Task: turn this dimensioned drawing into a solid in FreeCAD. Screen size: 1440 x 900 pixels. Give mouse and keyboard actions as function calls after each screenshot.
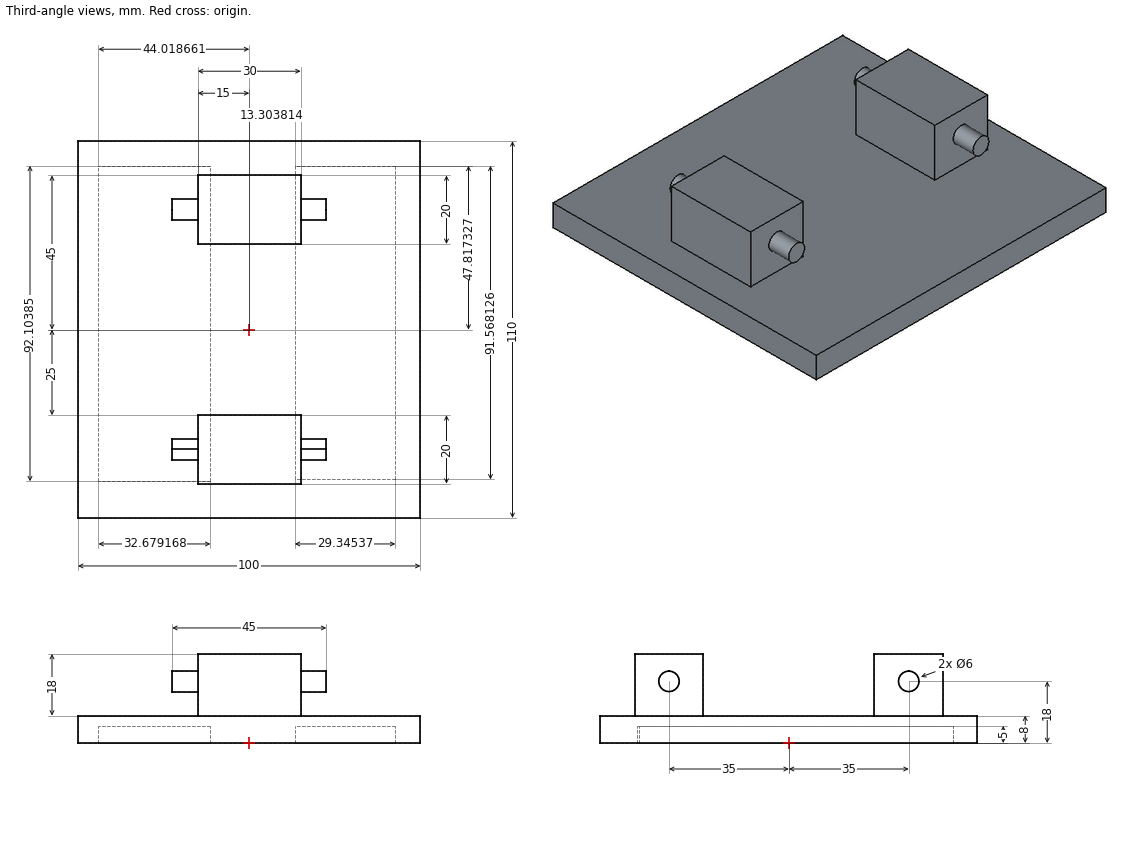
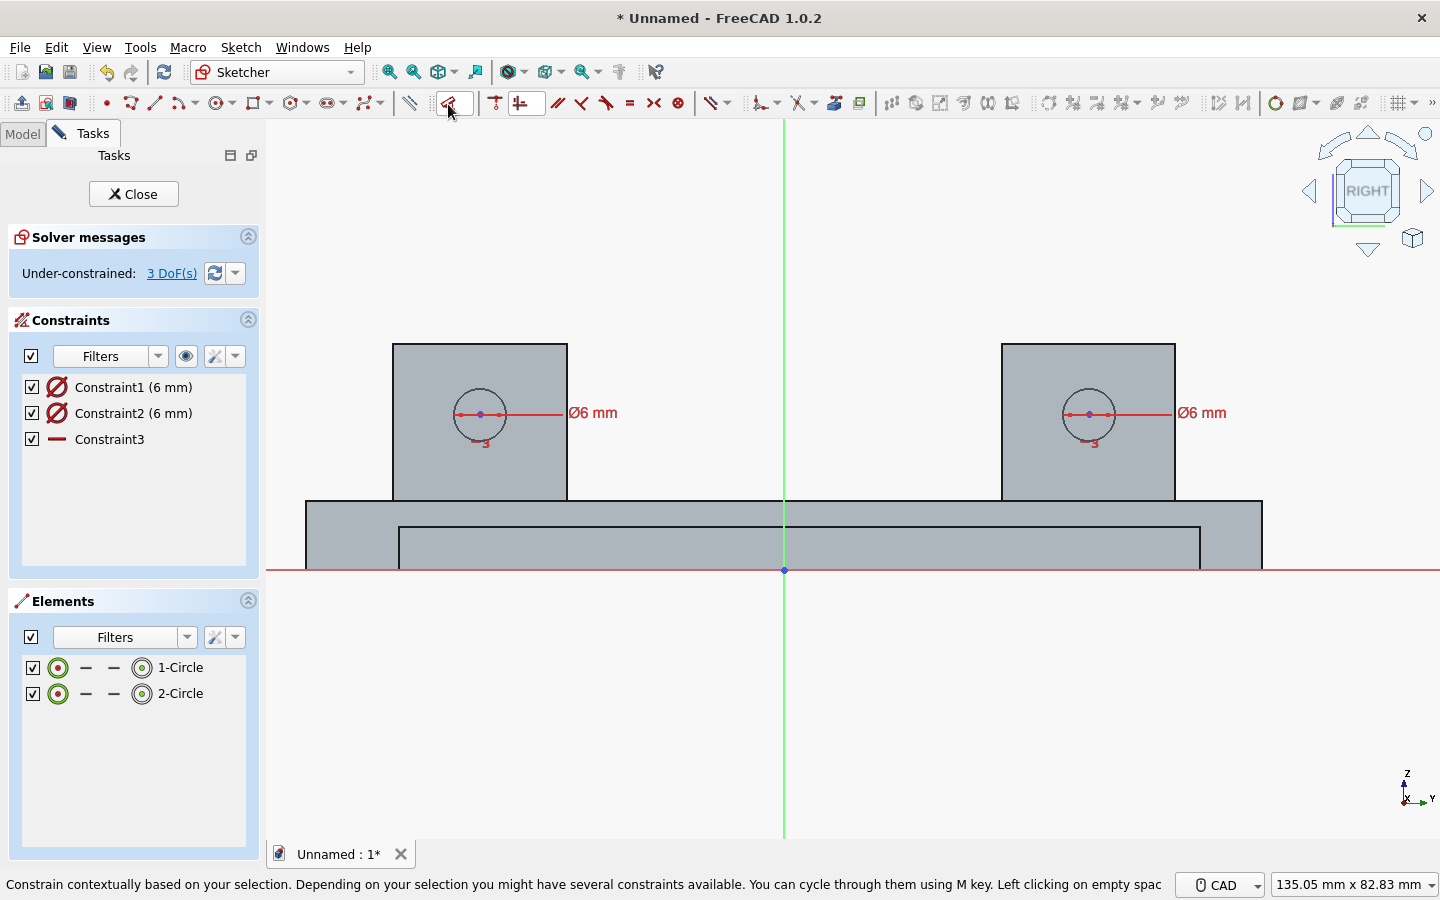
click(1089, 415)
click(937, 604)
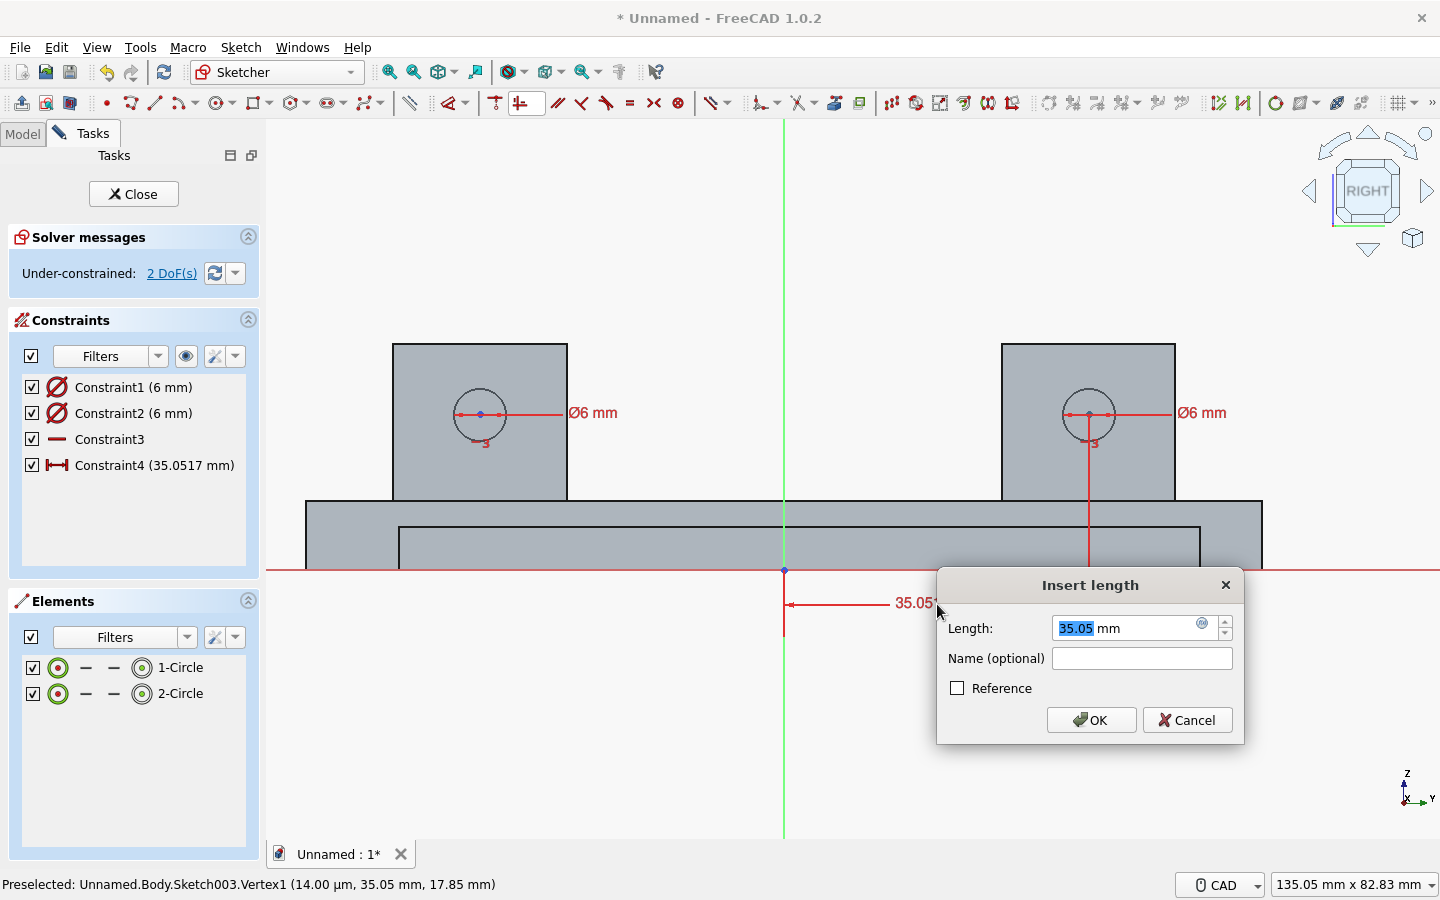
text(35)
key(Return)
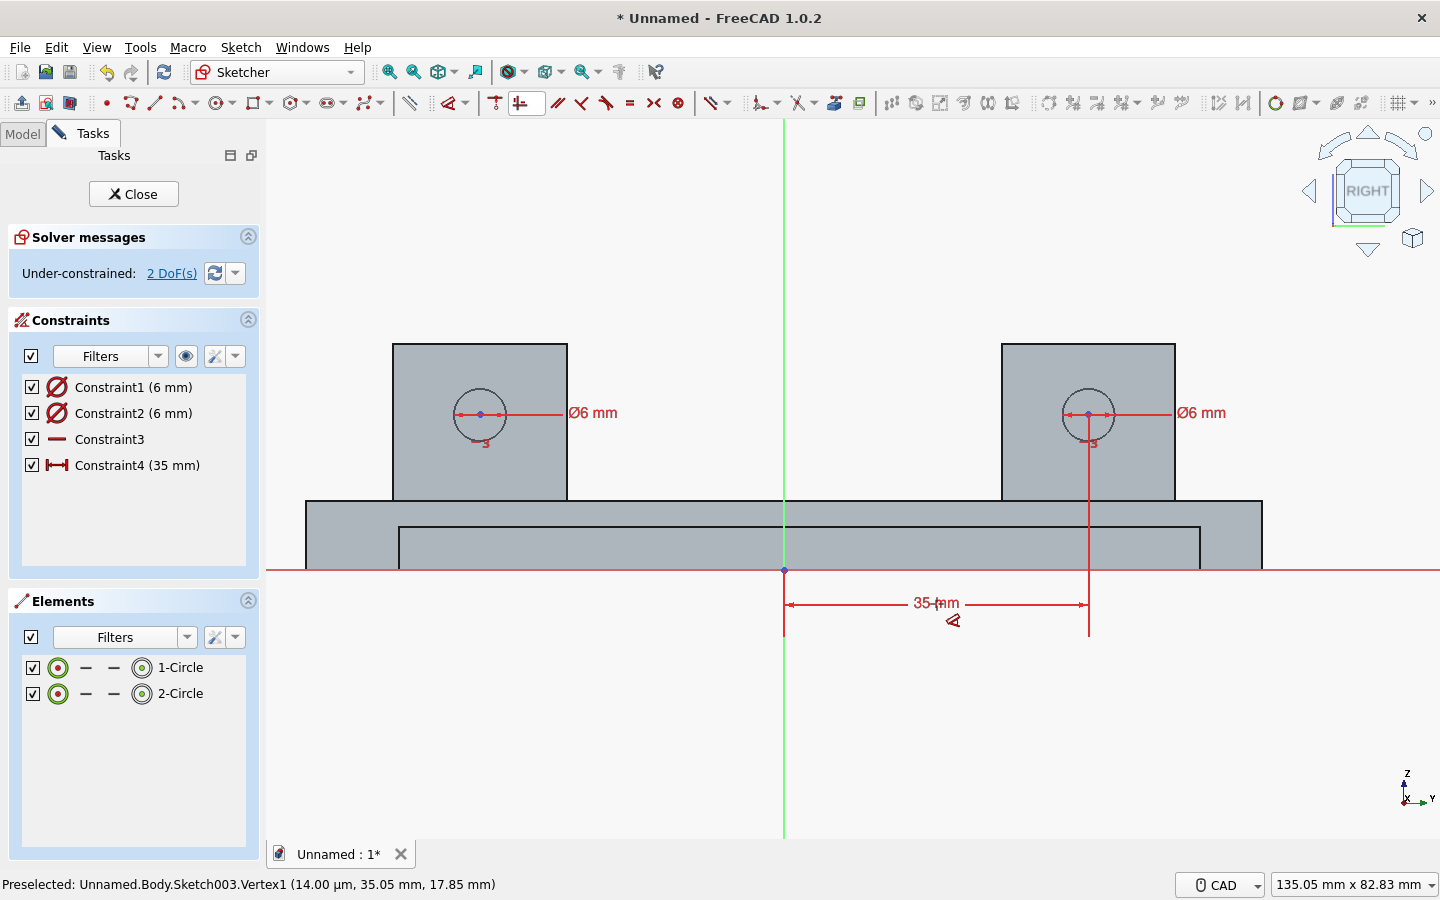
click(1089, 415)
click(1123, 493)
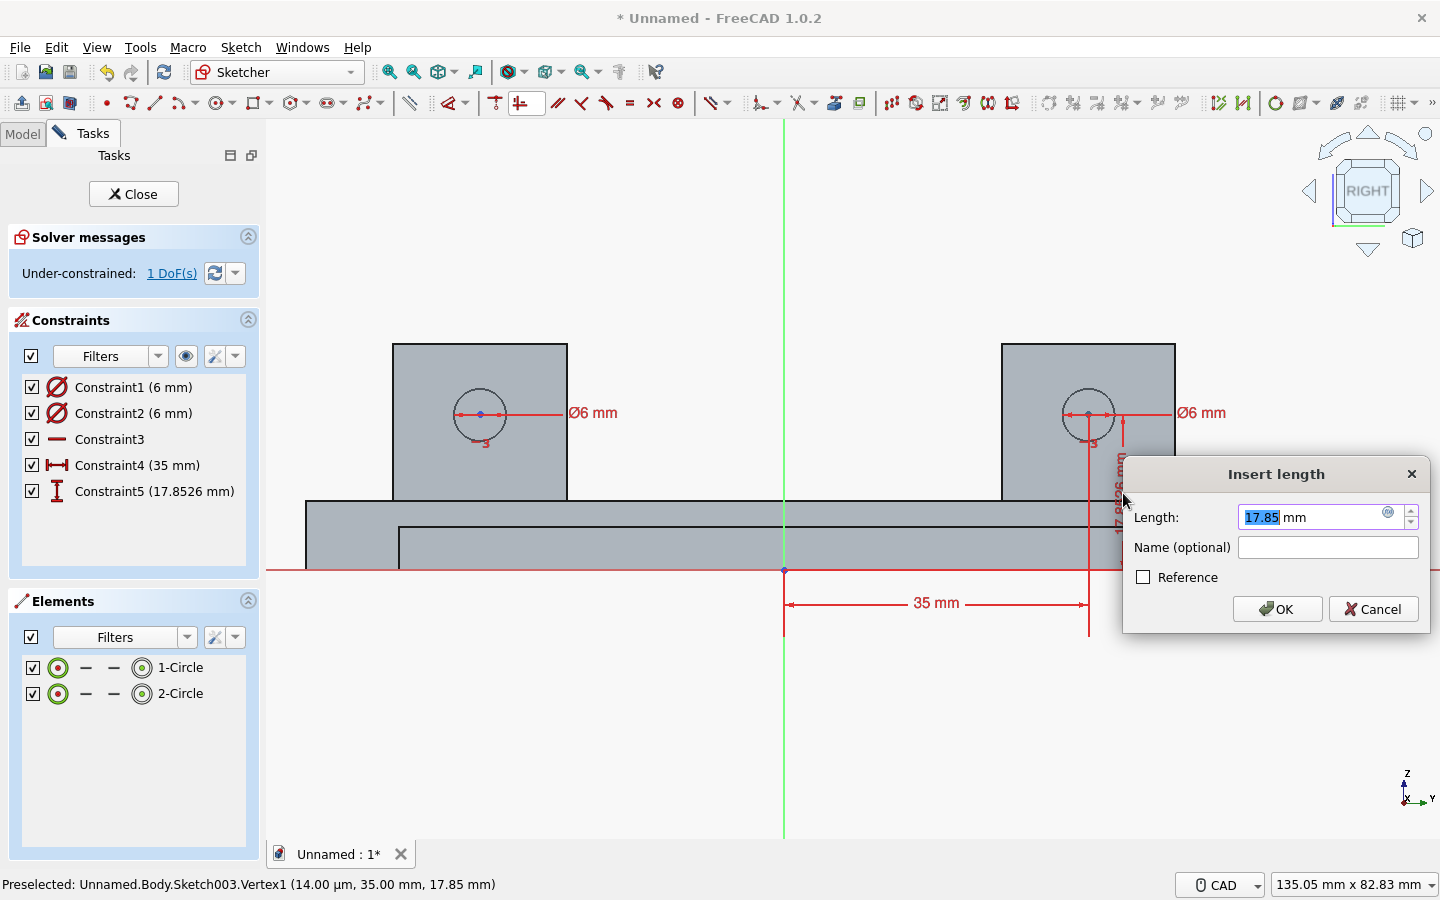
text(18)
key(Return)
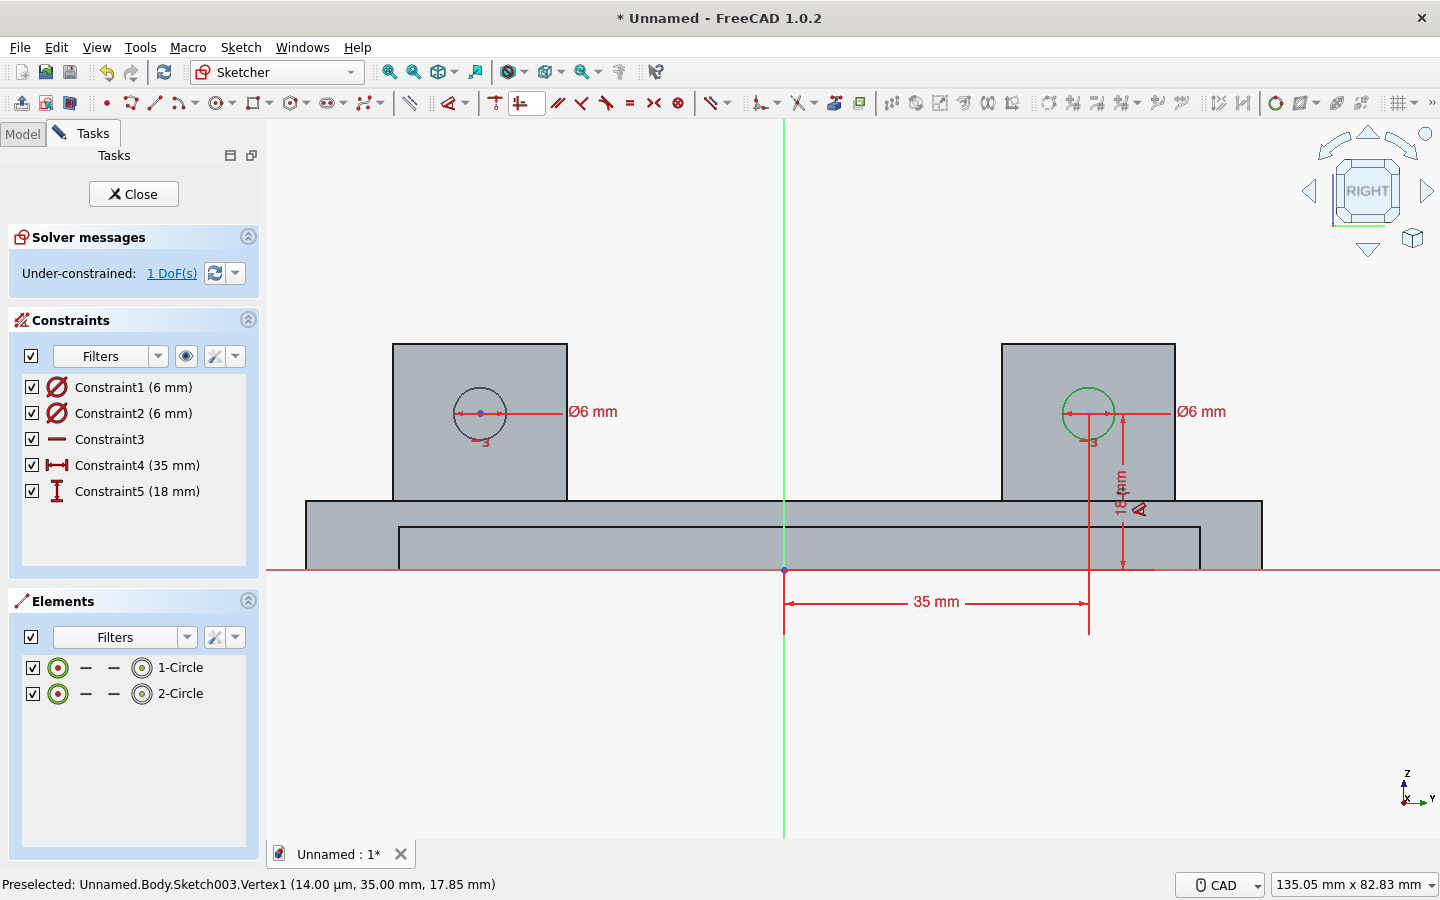
click(480, 414)
click(632, 604)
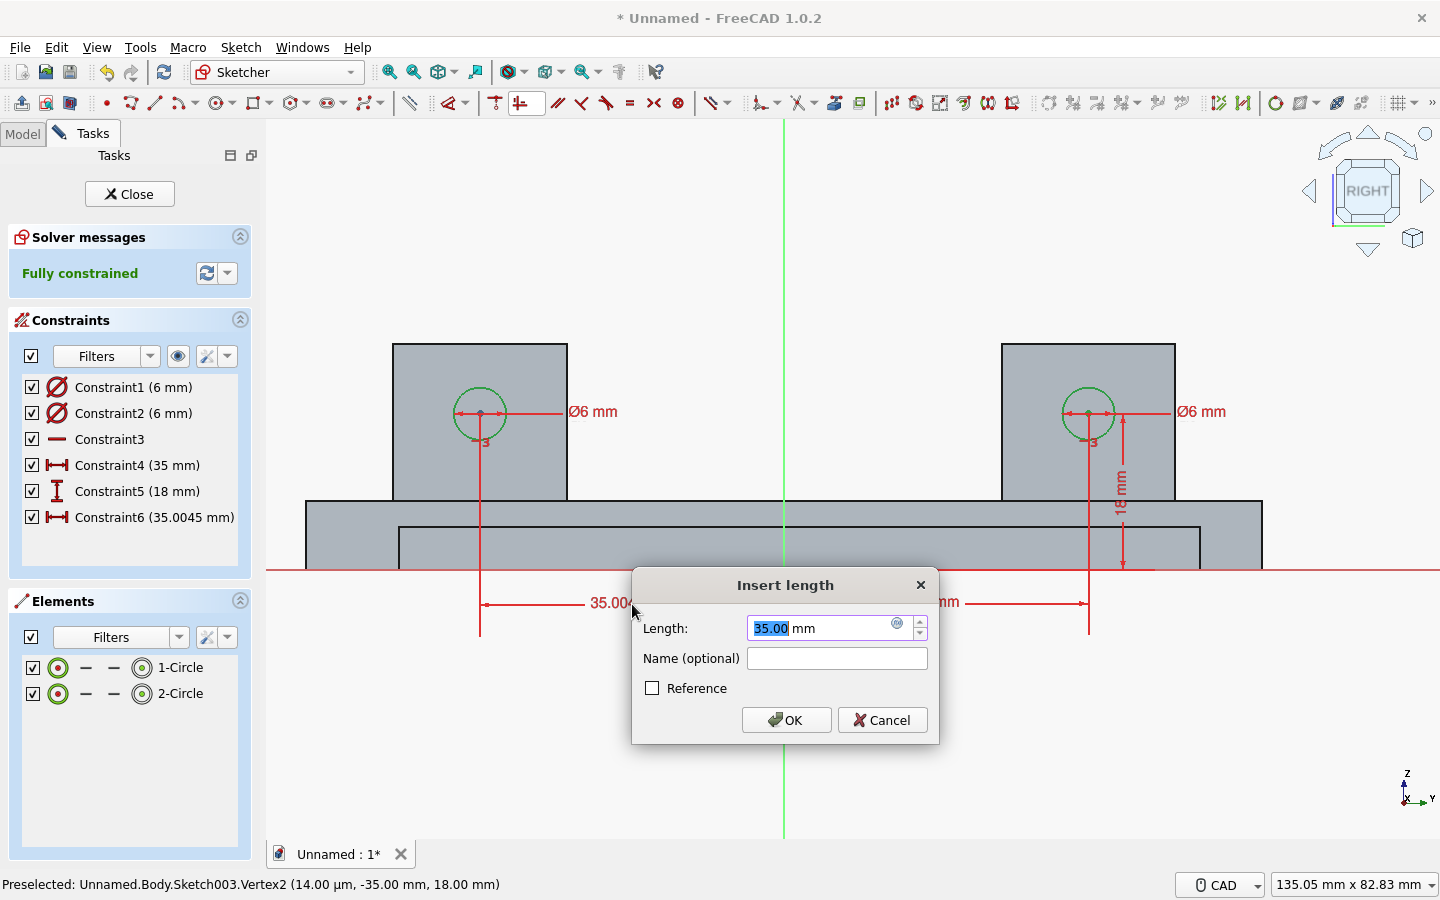
text(35)
key(Return)
key(Escape)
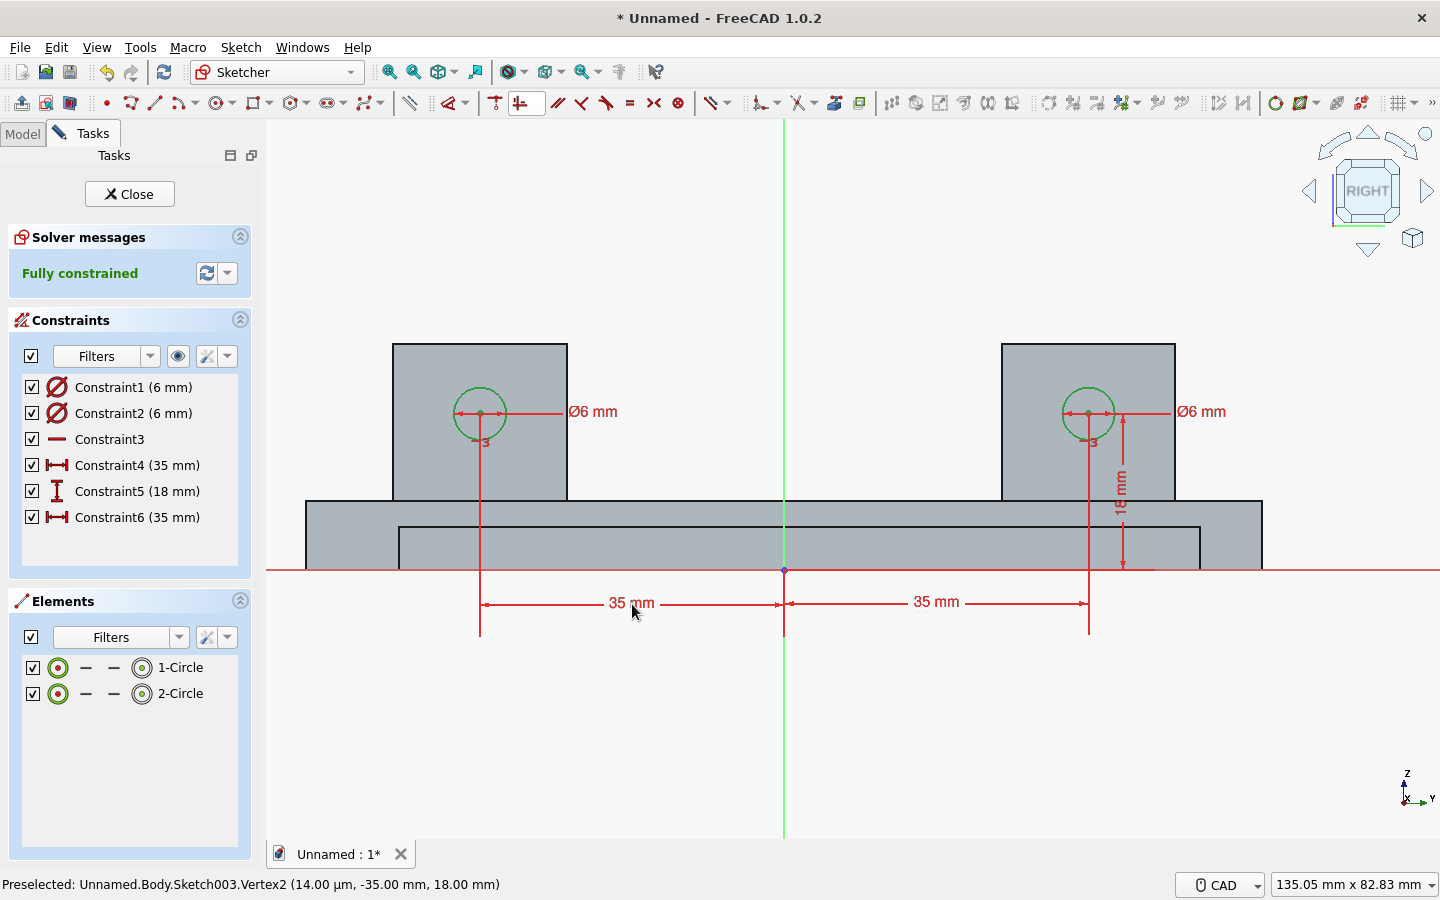
click(130, 194)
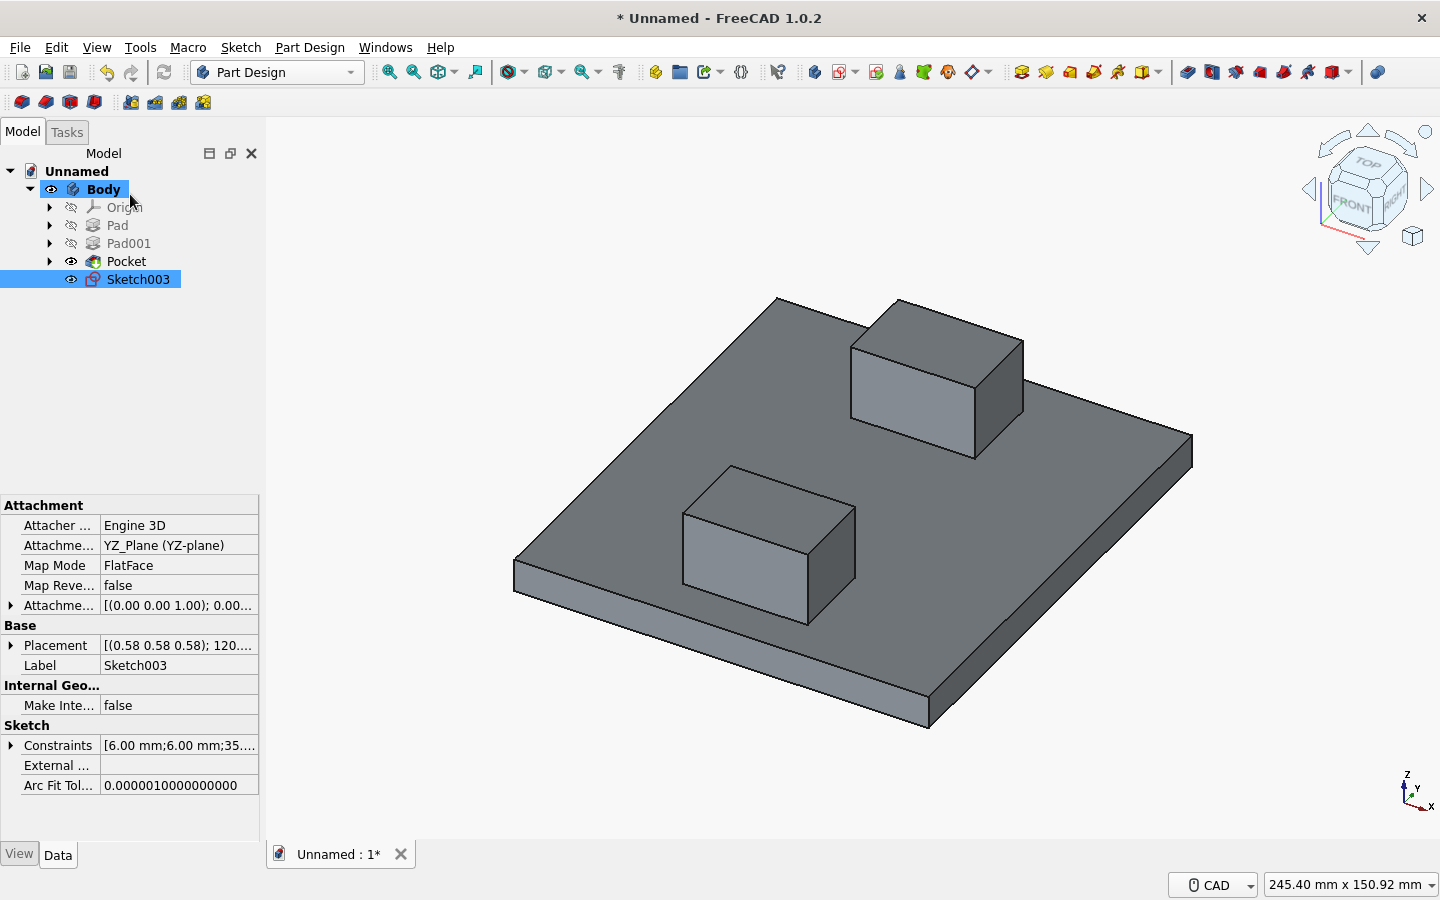
click(1022, 72)